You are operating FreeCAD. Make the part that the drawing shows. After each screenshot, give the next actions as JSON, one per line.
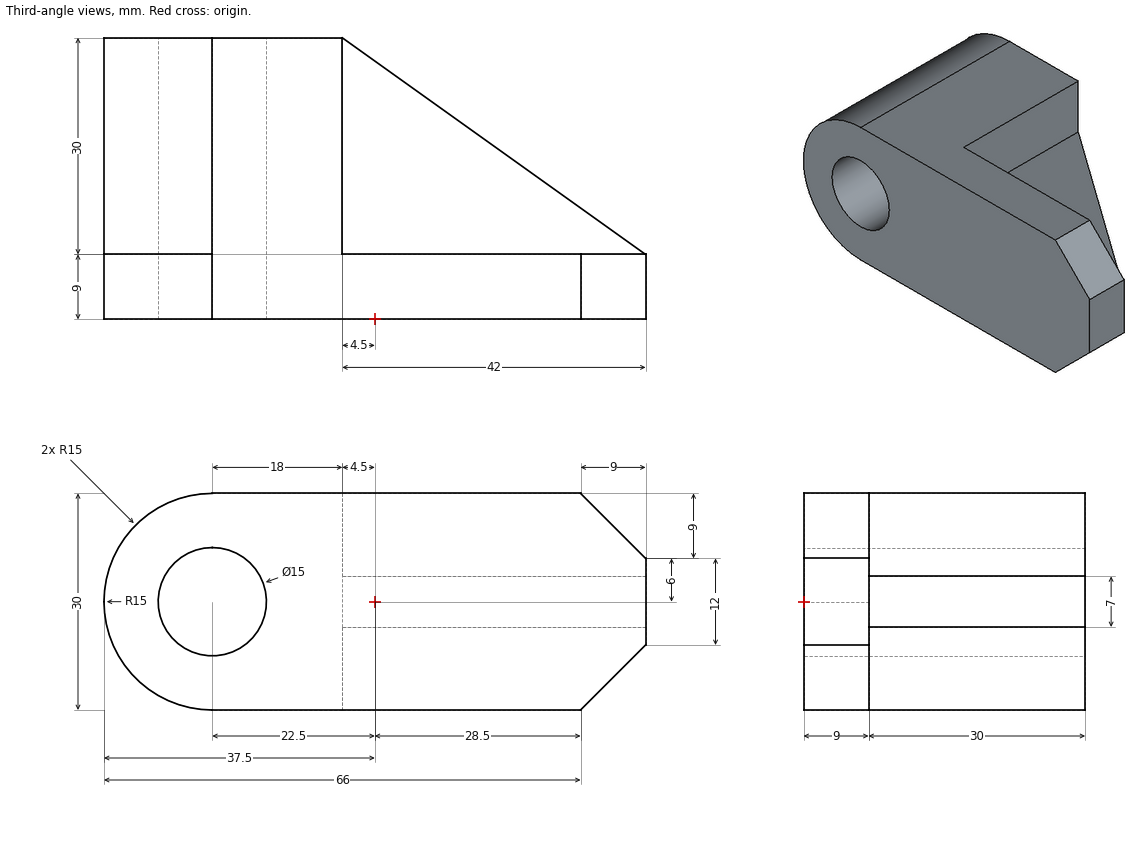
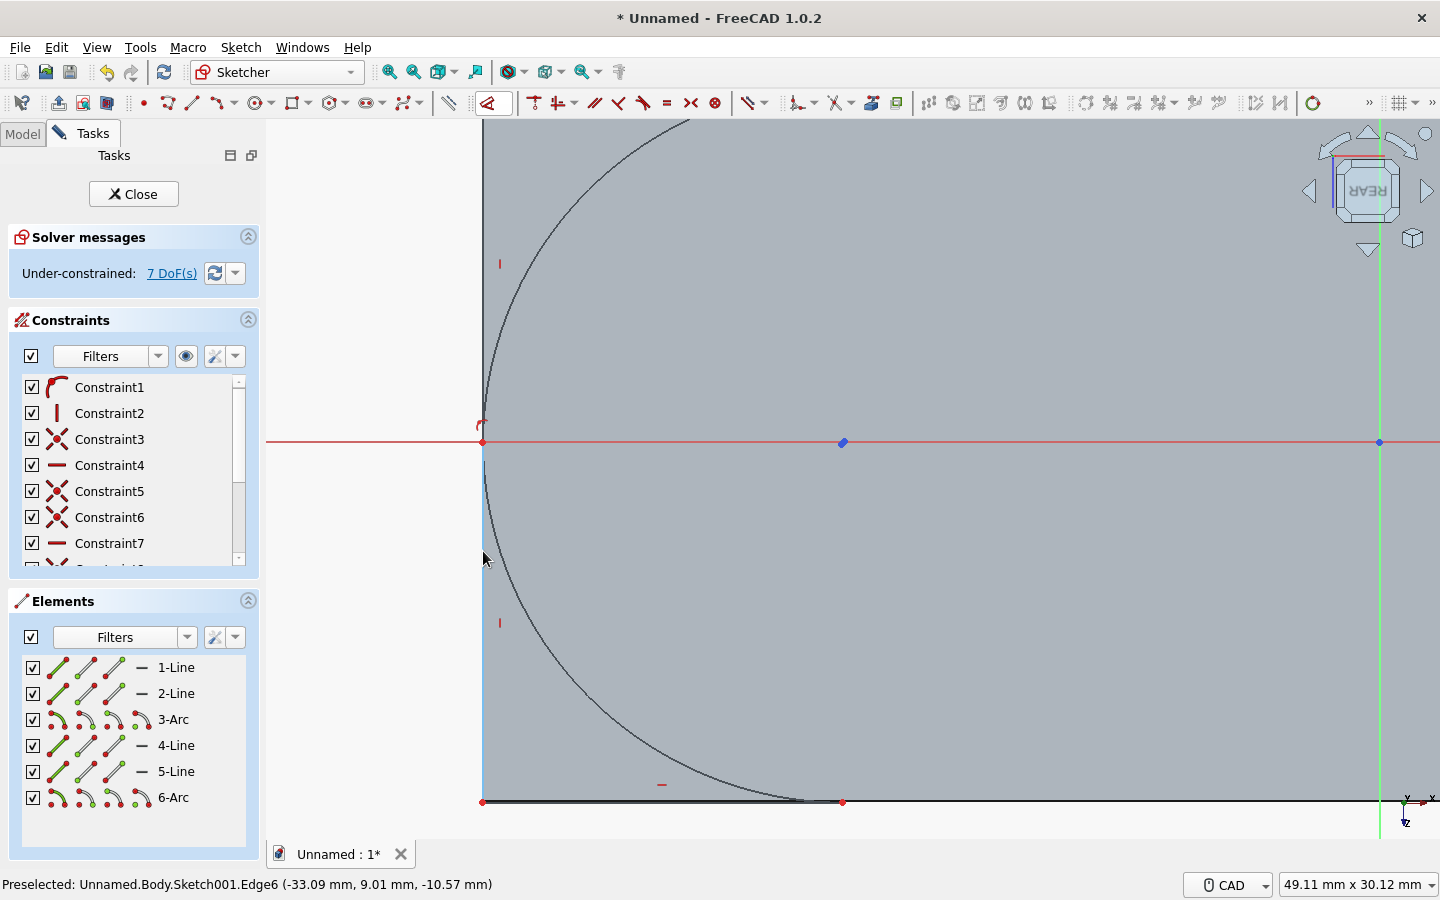
{"action": "left_click", "coordinate": [483, 551]}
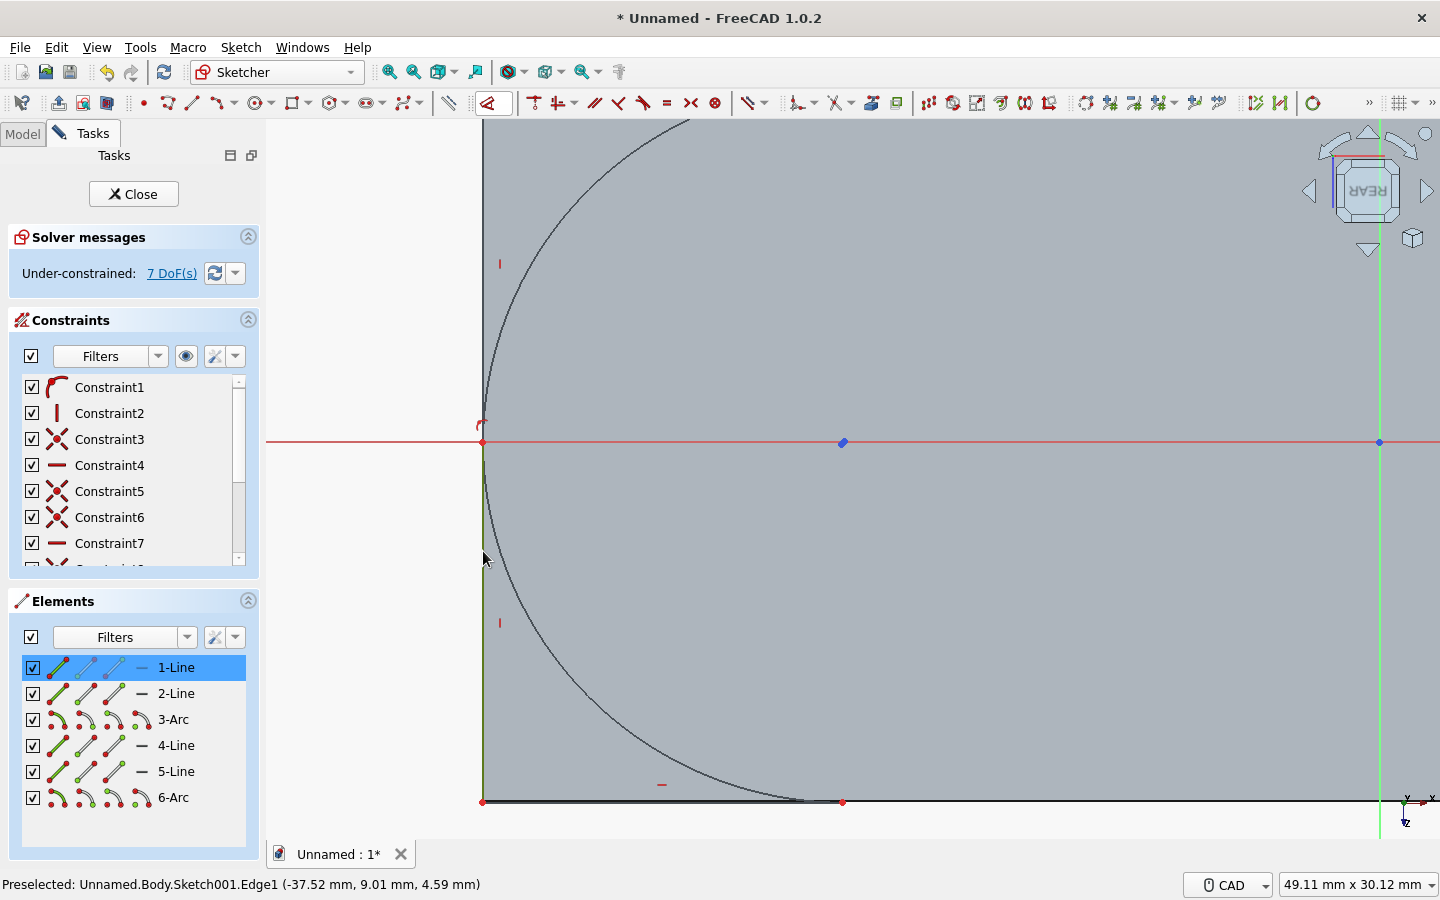
{"action": "left_click", "coordinate": [522, 606]}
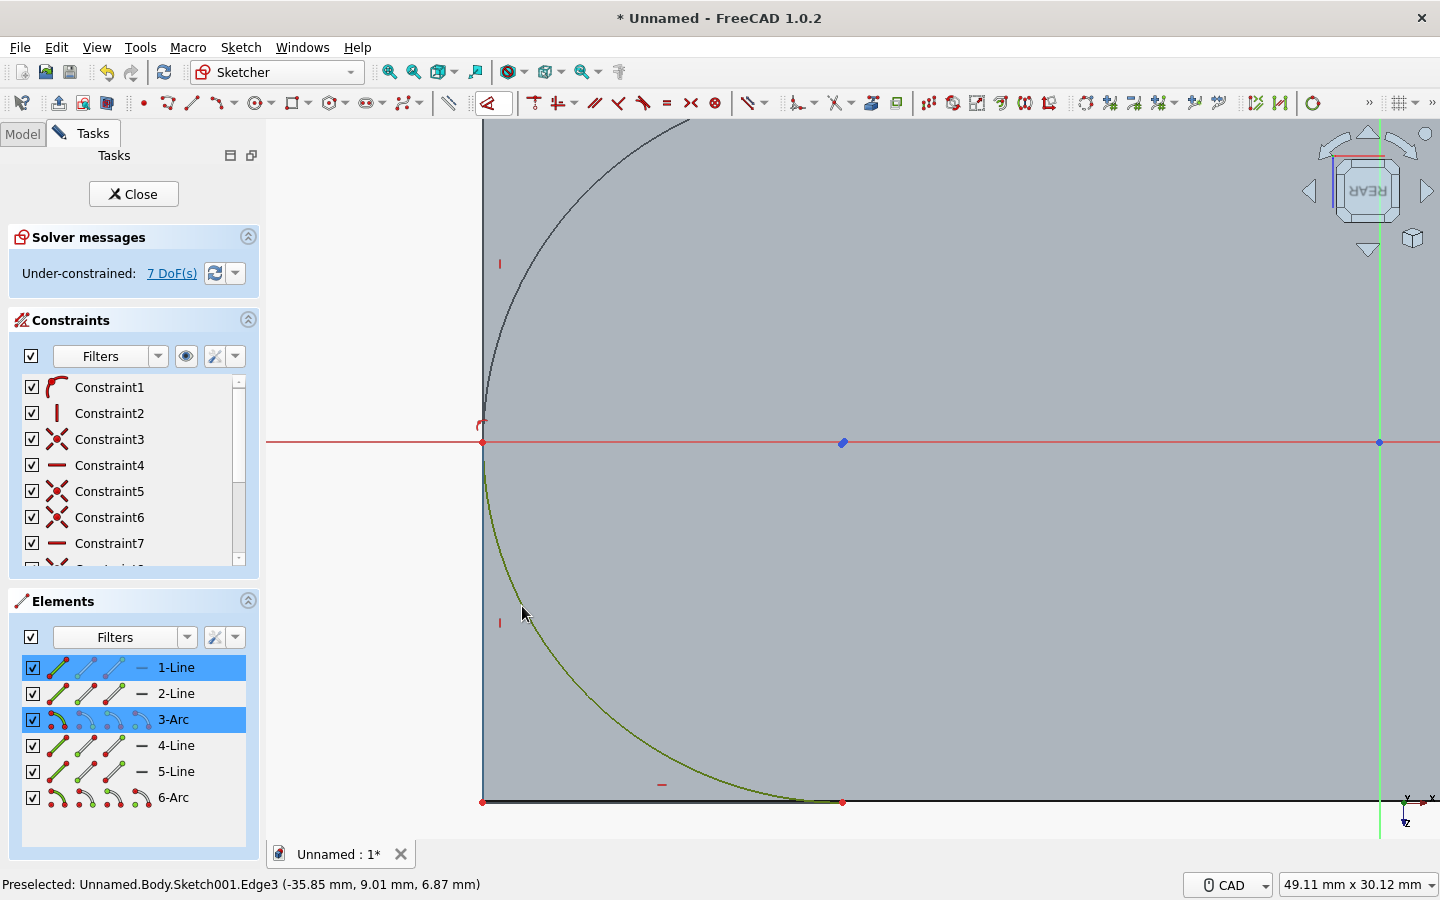
{"action": "key", "text": "t"}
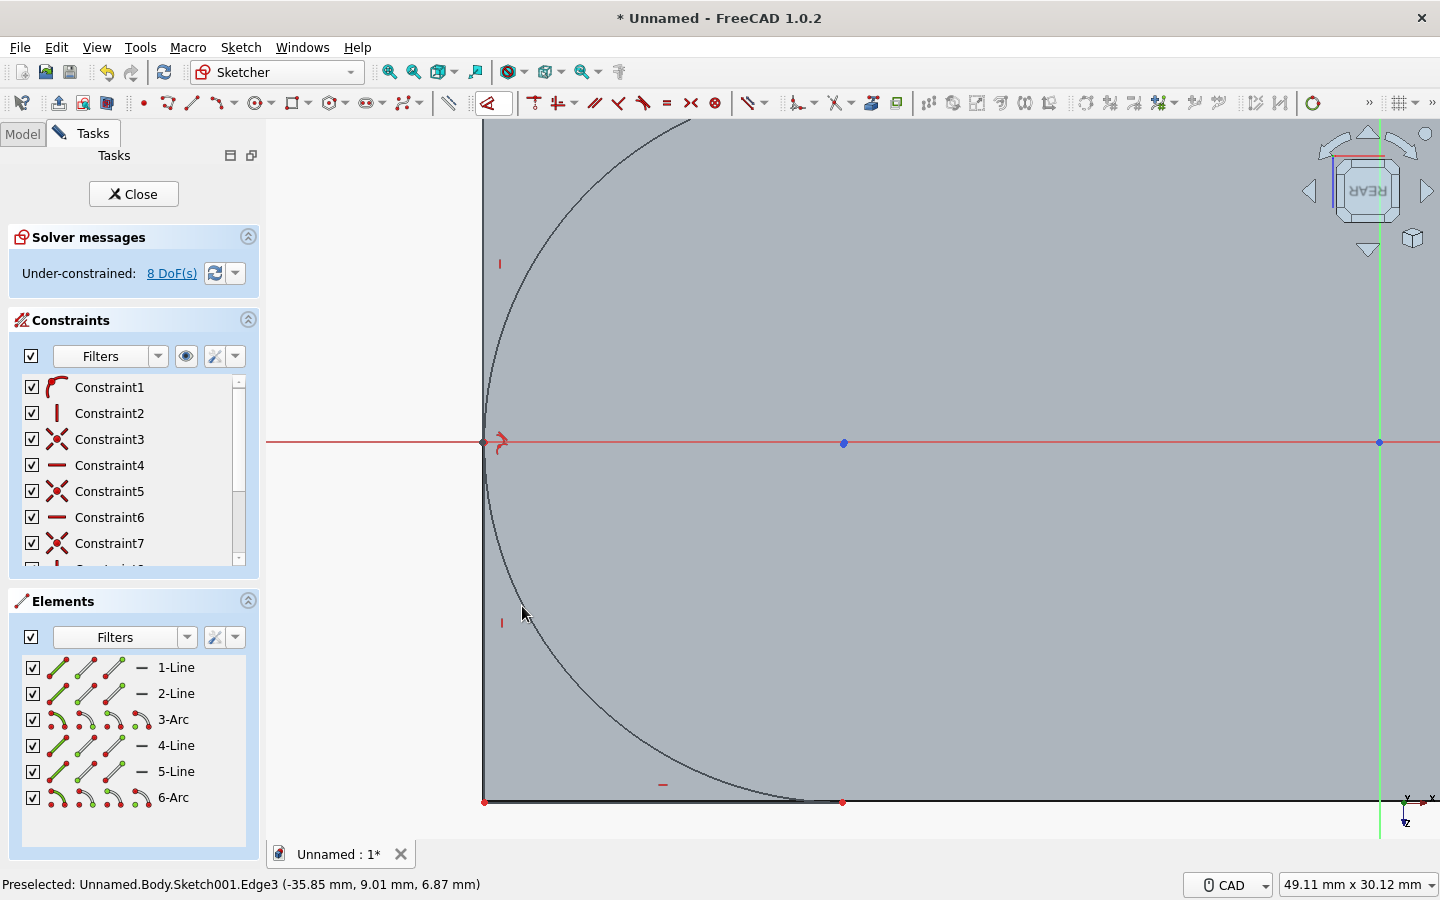
{"action": "left_click", "coordinate": [484, 551]}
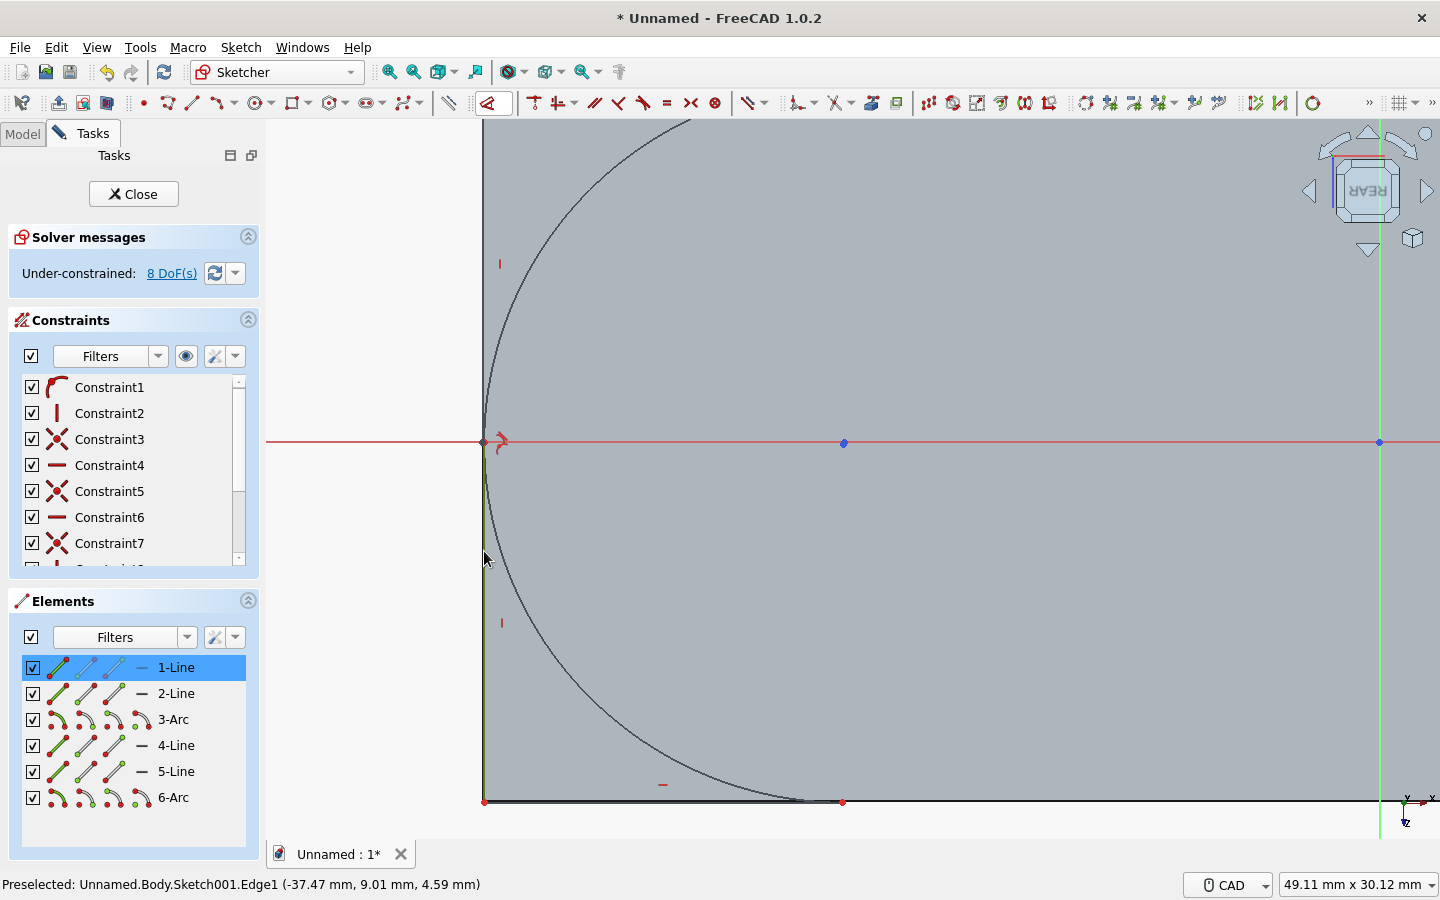
{"action": "left_click", "coordinate": [524, 280]}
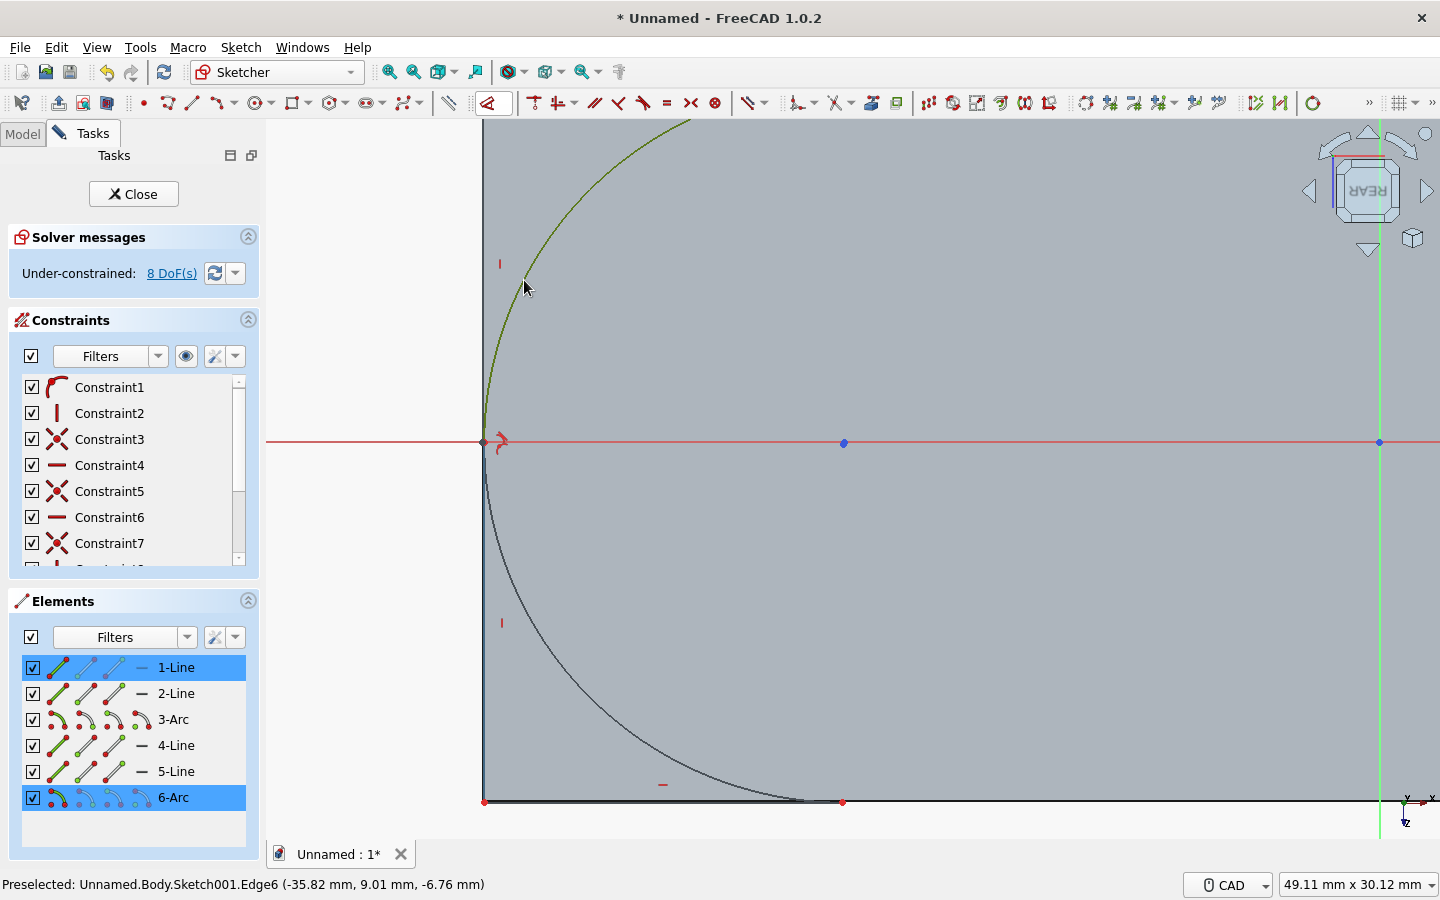
{"action": "left_click", "coordinate": [644, 104]}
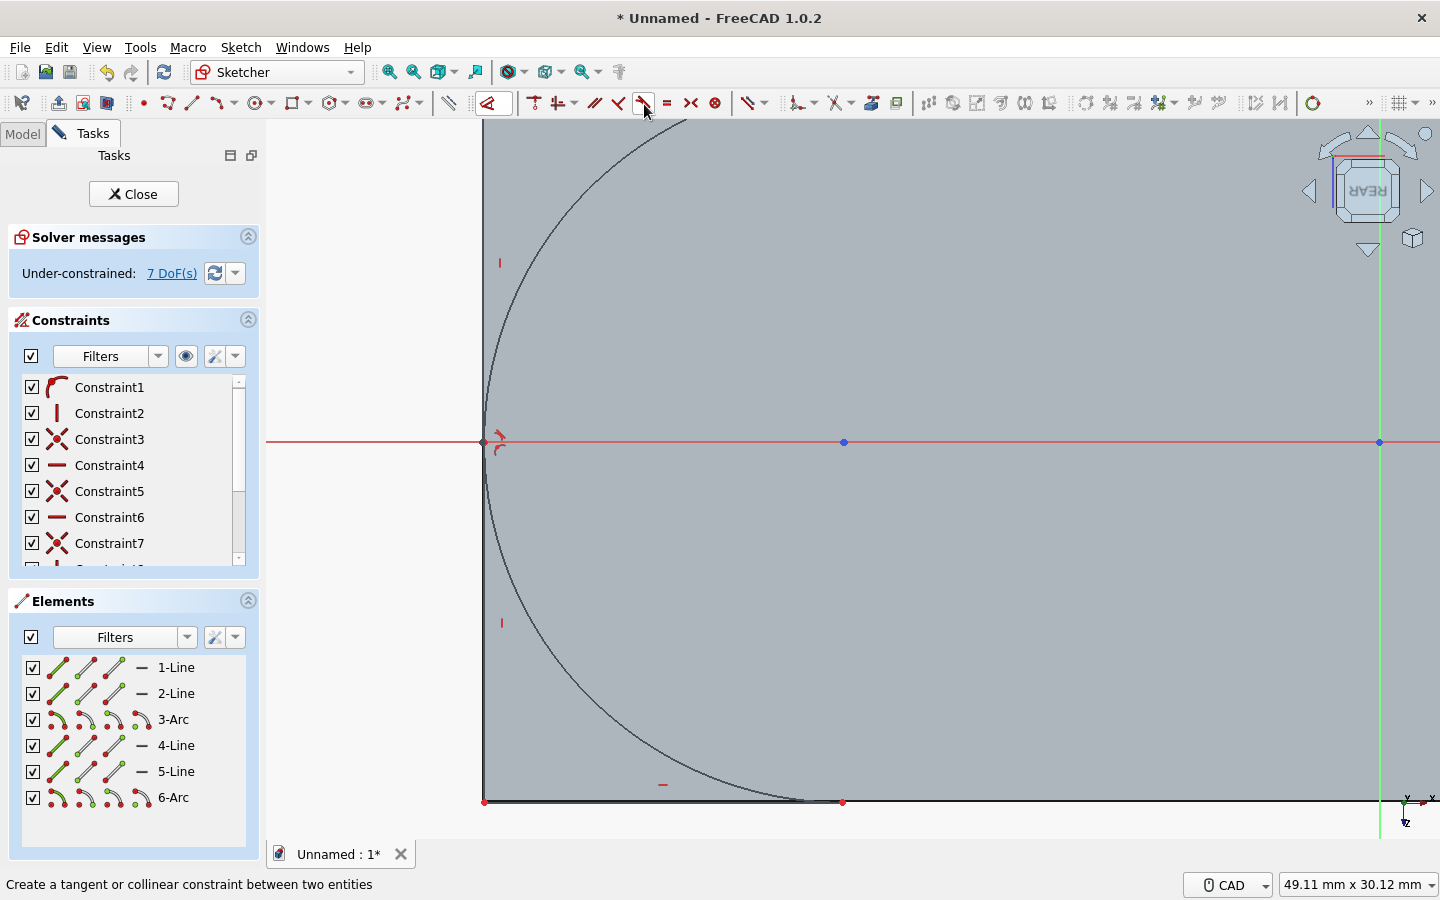
{"action": "left_click", "coordinate": [592, 803]}